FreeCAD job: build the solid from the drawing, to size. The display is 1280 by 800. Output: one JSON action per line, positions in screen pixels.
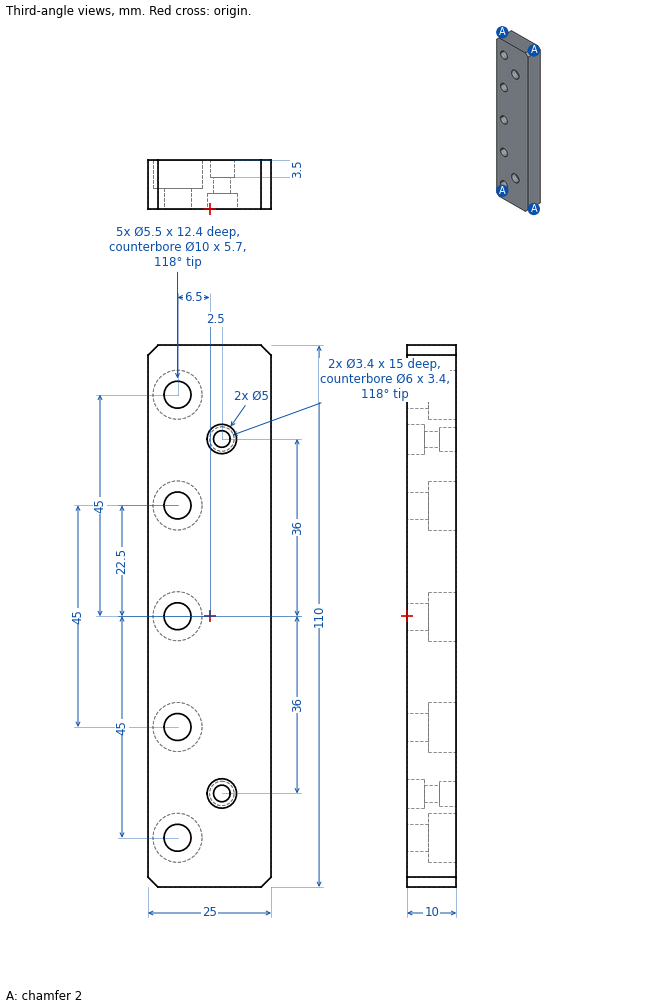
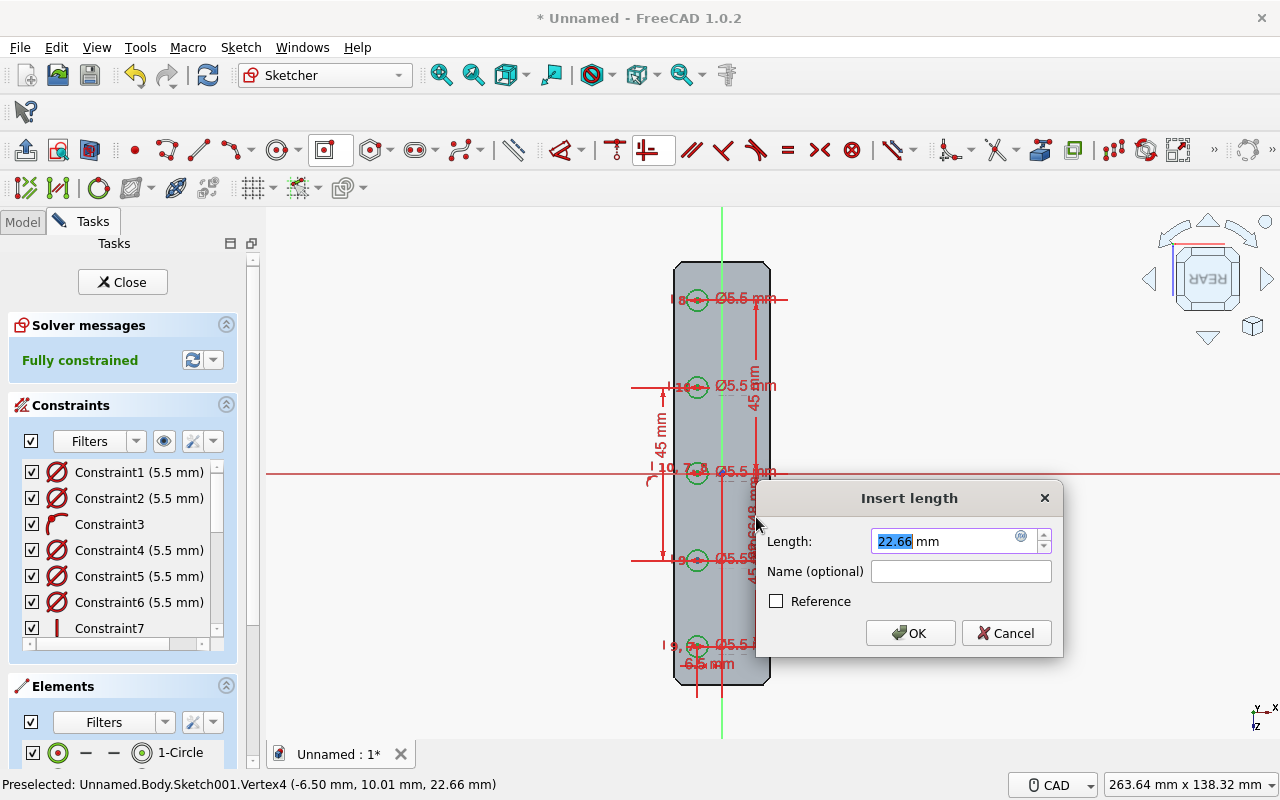
{"action": "type", "text": "22.5"}
{"action": "key", "text": "Return"}
{"action": "key", "text": "Escape"}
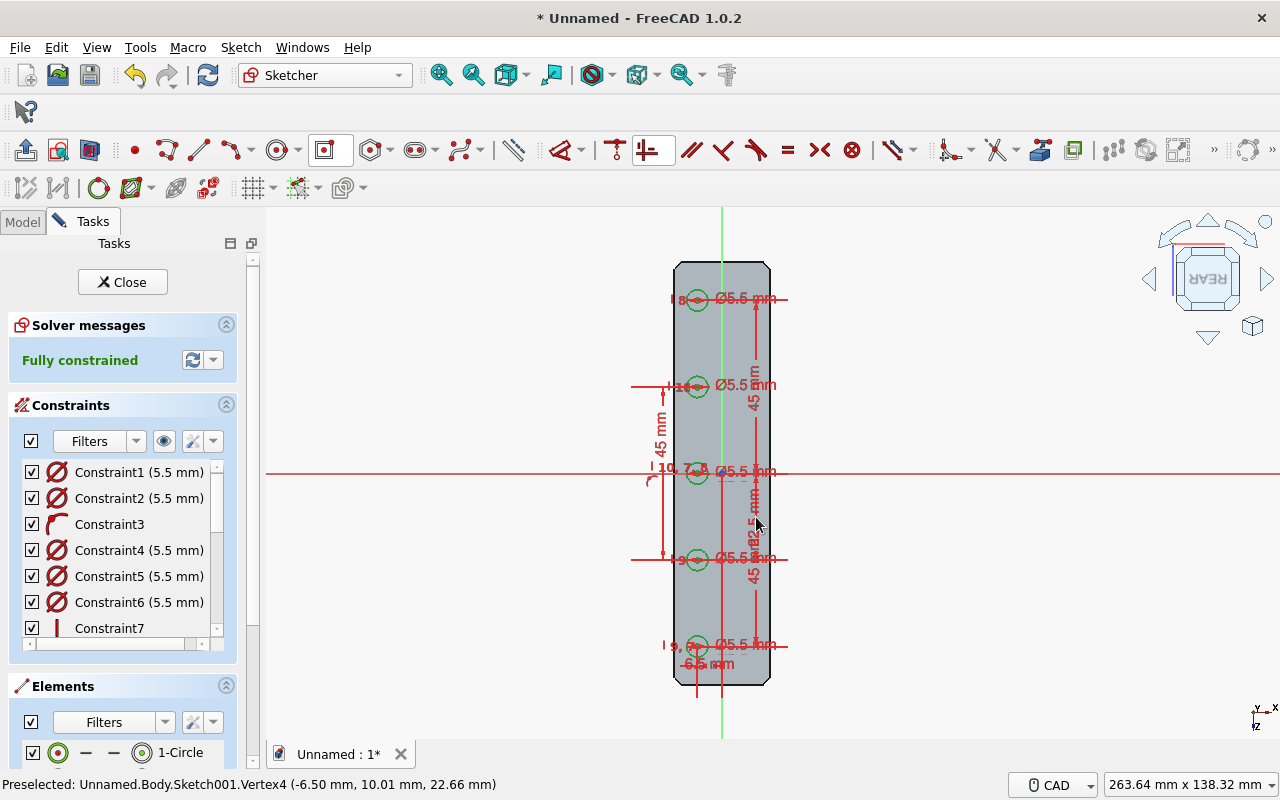
{"action": "left_click", "coordinate": [123, 282]}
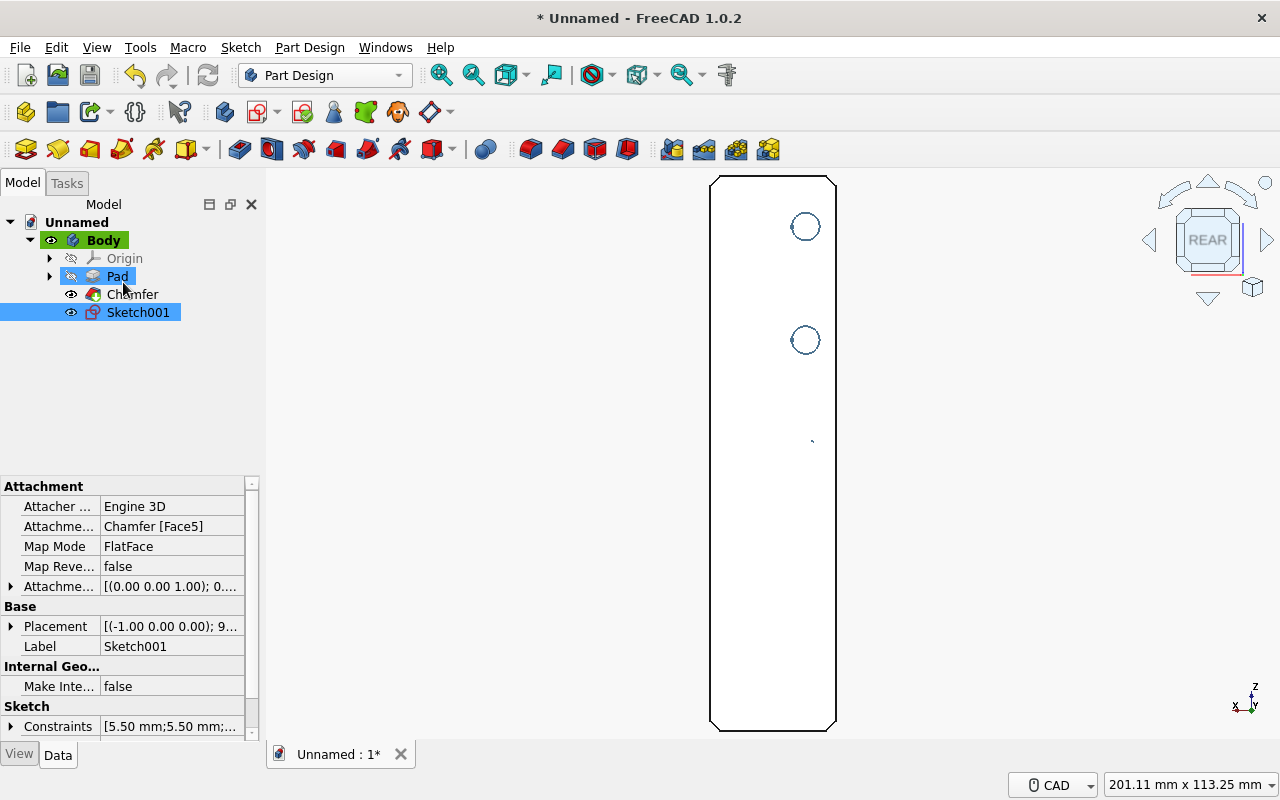
{"action": "left_click", "coordinate": [272, 150]}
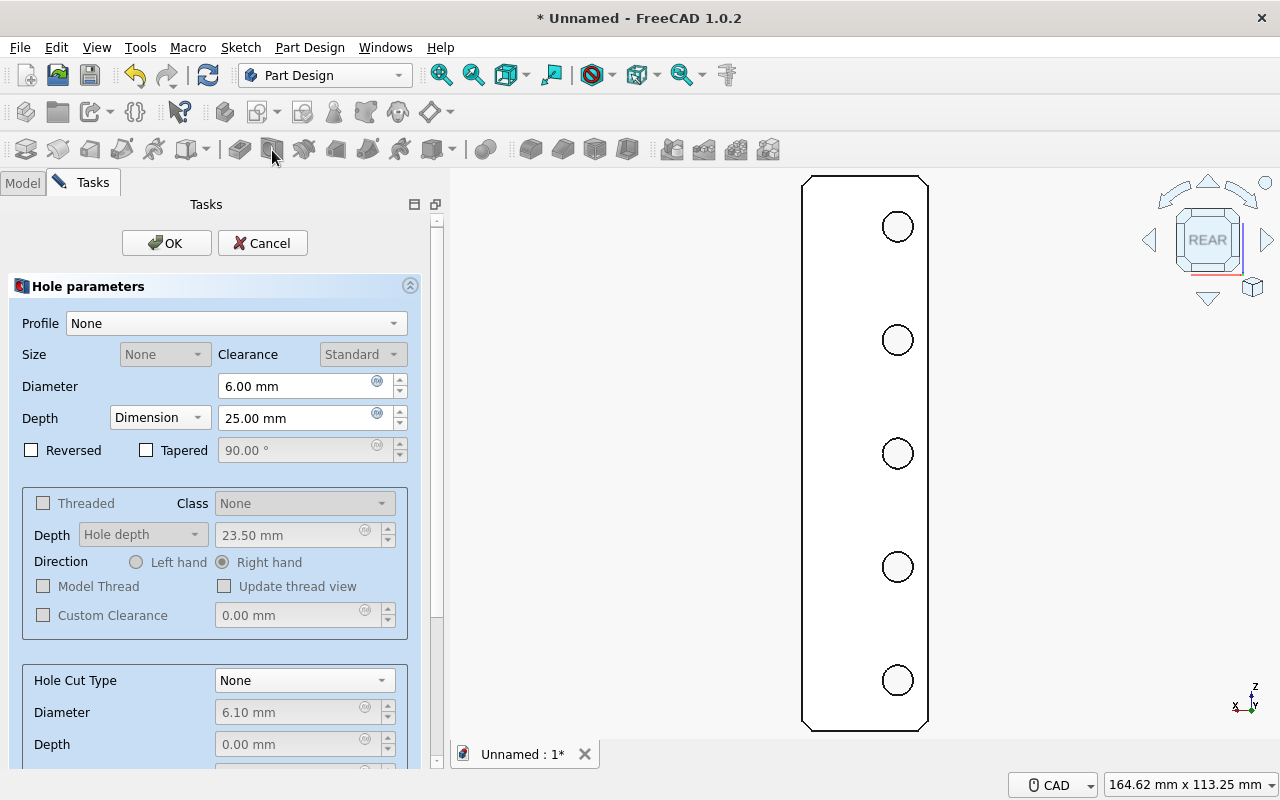
{"action": "triple_click", "coordinate": [305, 386]}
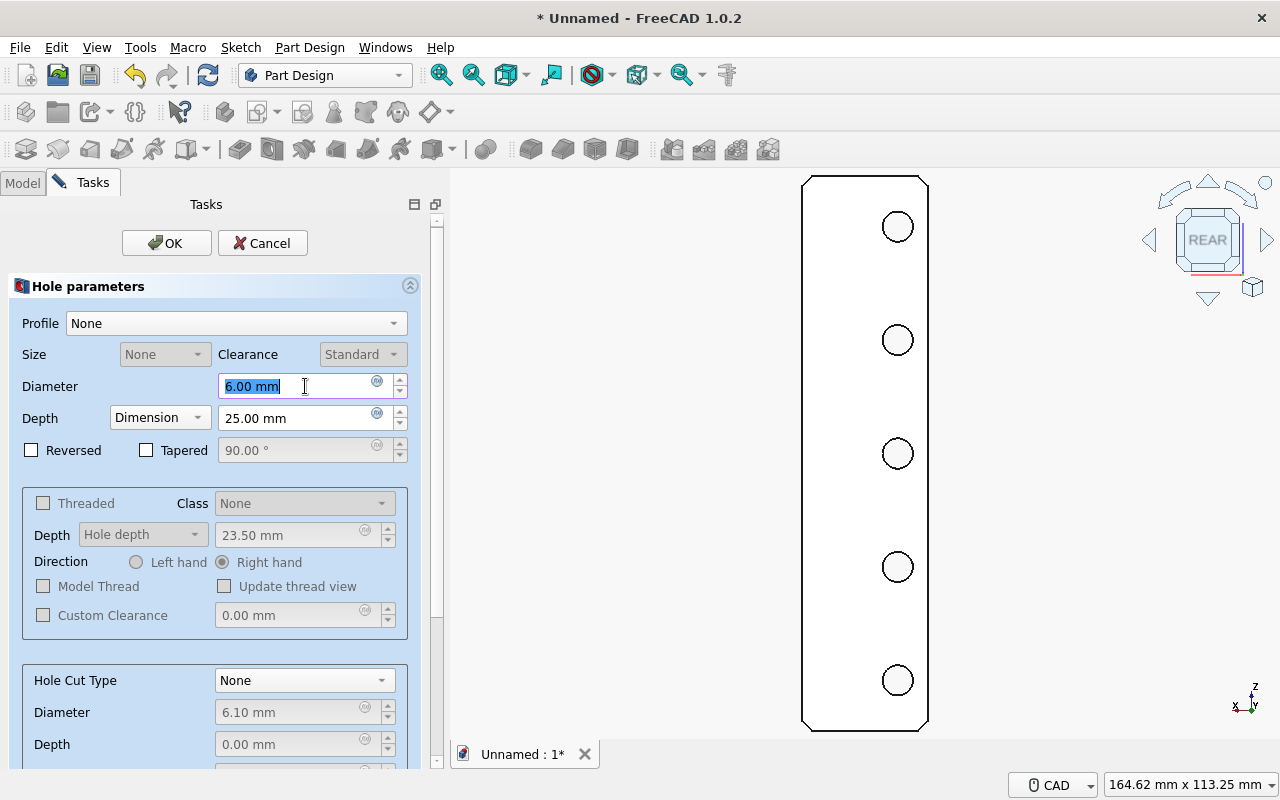
{"action": "type", "text": "5.5"}
{"action": "key", "text": "Tab"}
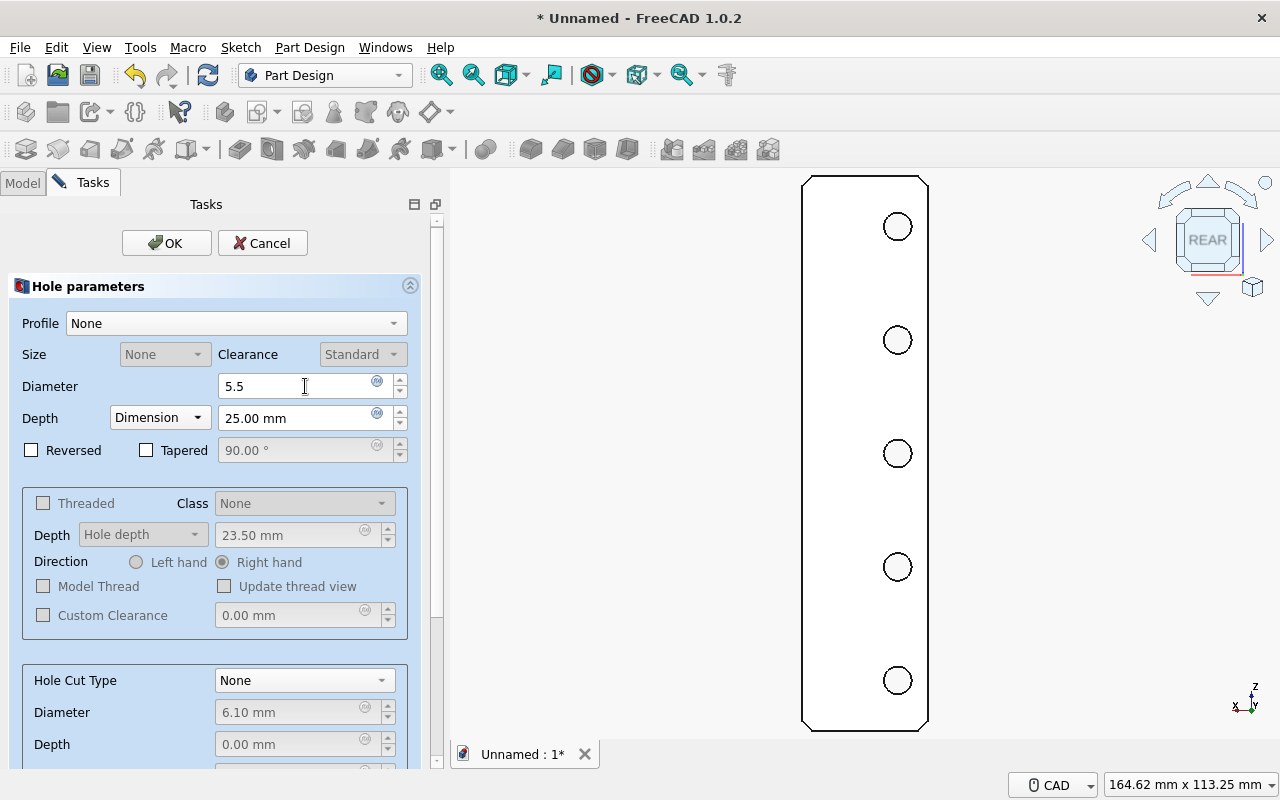
{"action": "triple_click", "coordinate": [305, 418]}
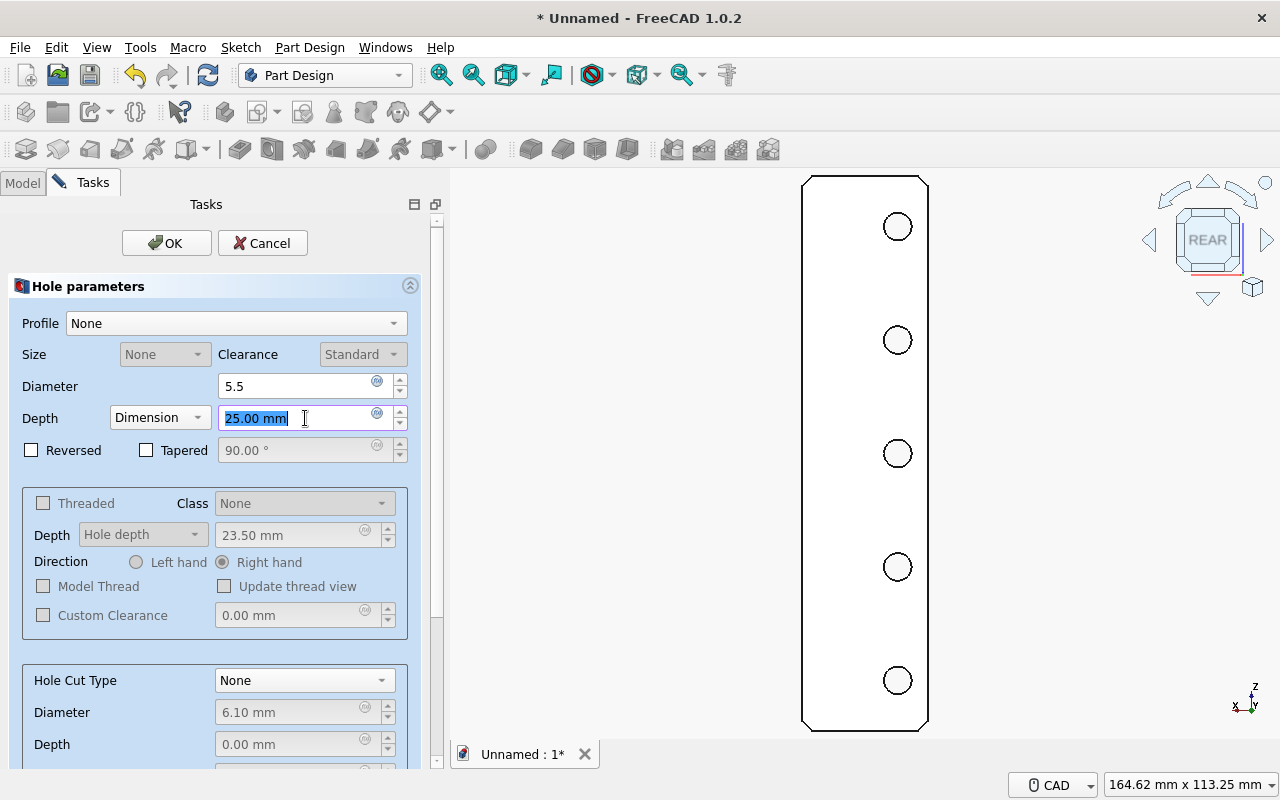
{"action": "type", "text": "12.4"}
{"action": "key", "text": "Tab"}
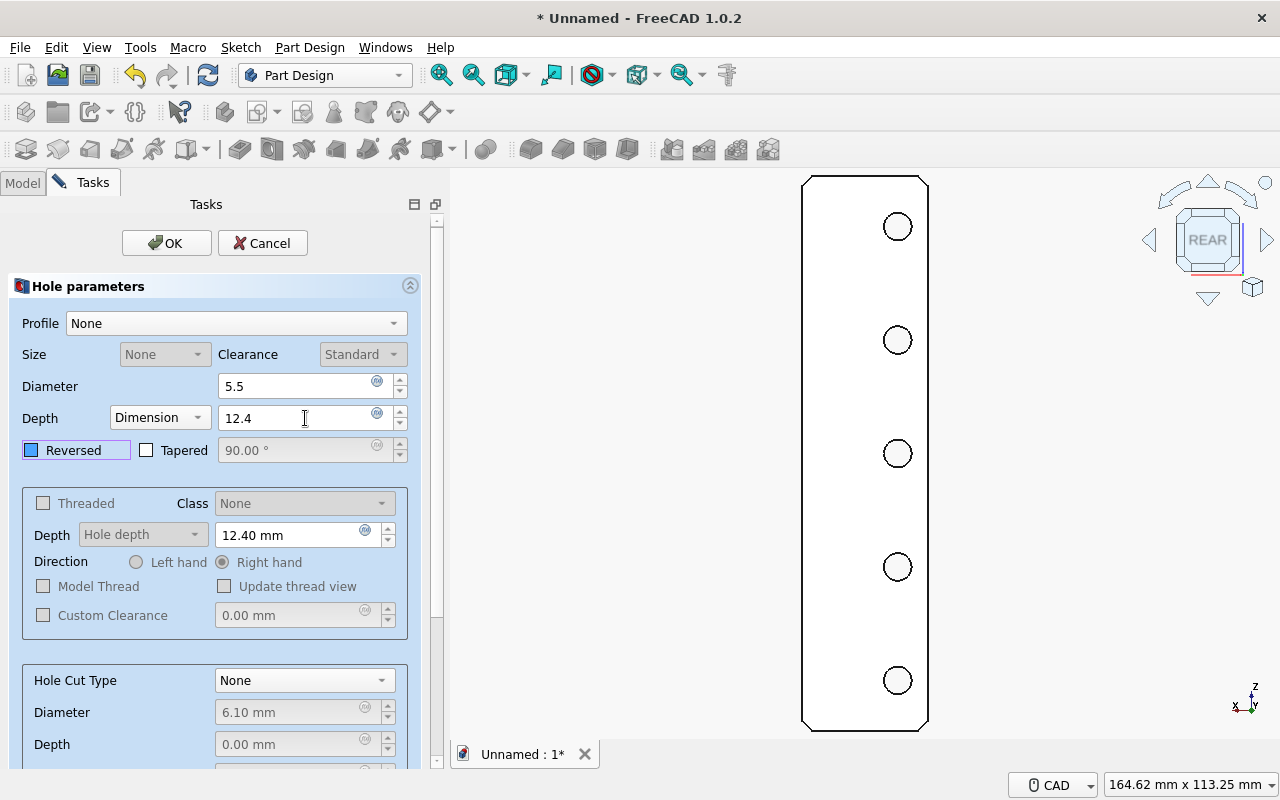
{"action": "left_click", "coordinate": [306, 680]}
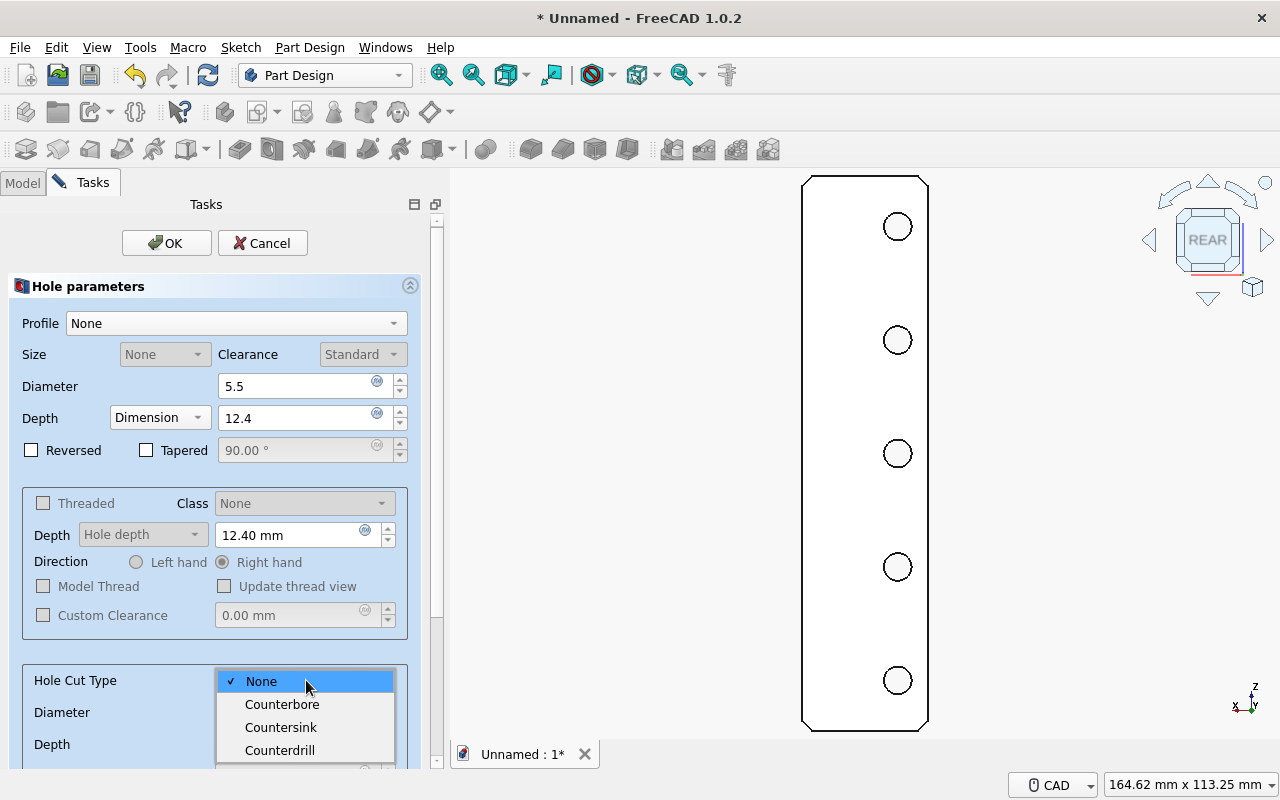
{"action": "left_click", "coordinate": [304, 704]}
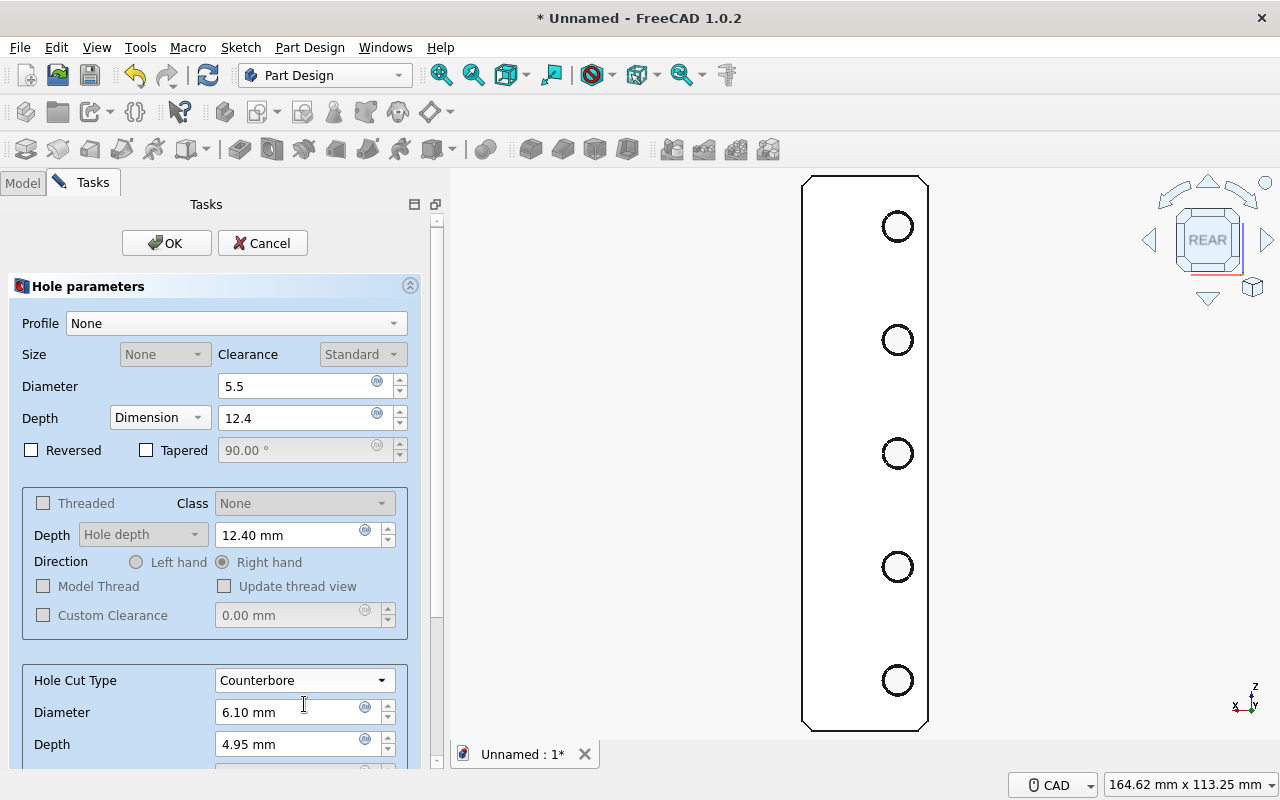
{"action": "triple_click", "coordinate": [298, 712]}